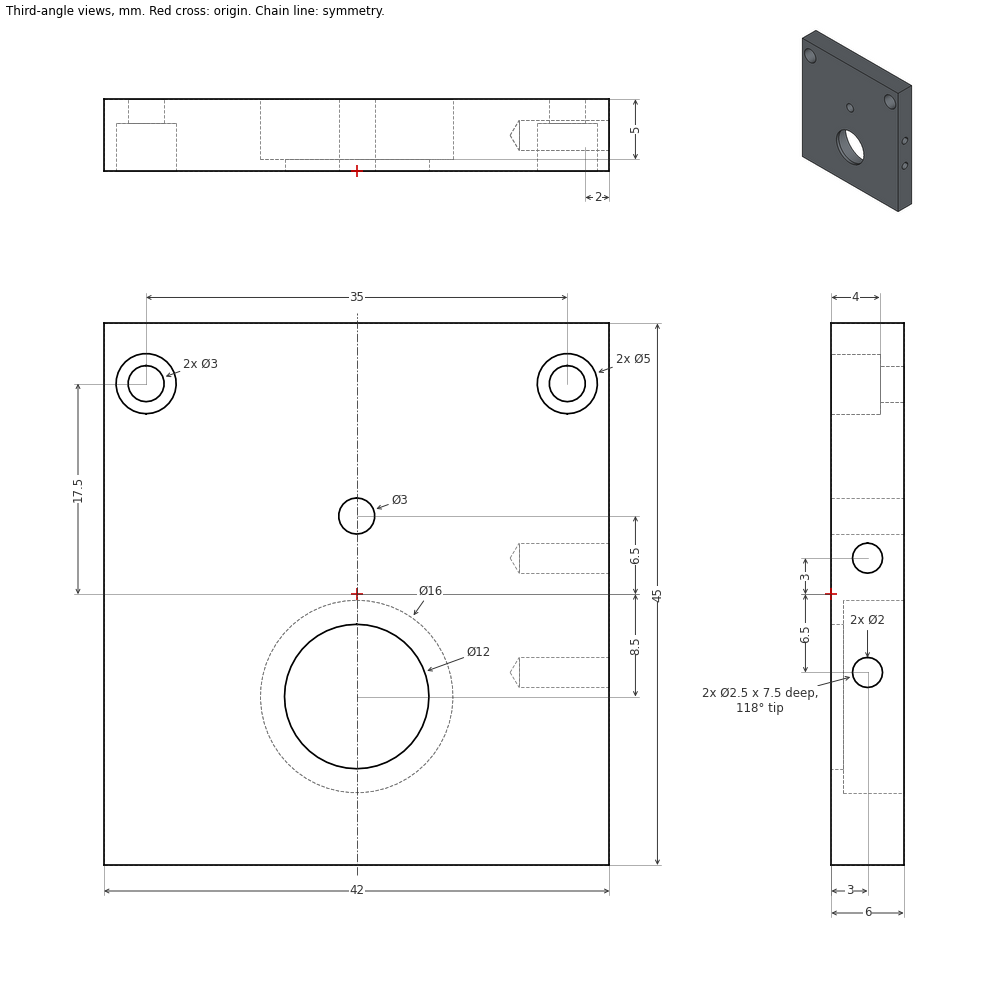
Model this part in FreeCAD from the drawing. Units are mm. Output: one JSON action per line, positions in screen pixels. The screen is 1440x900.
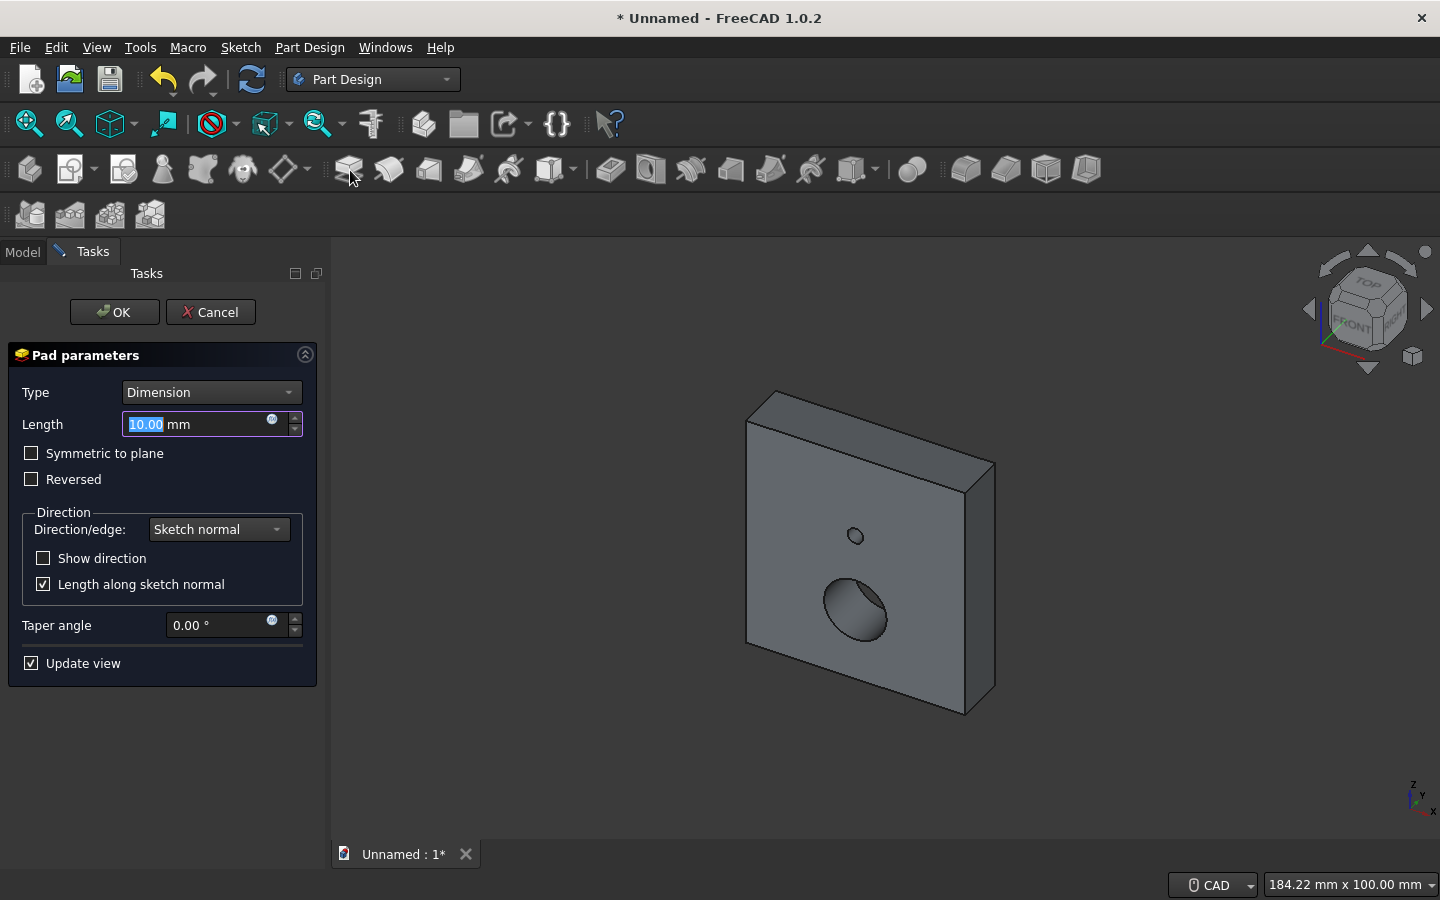
{"action": "type", "text": "6"}
{"action": "key", "text": "Tab"}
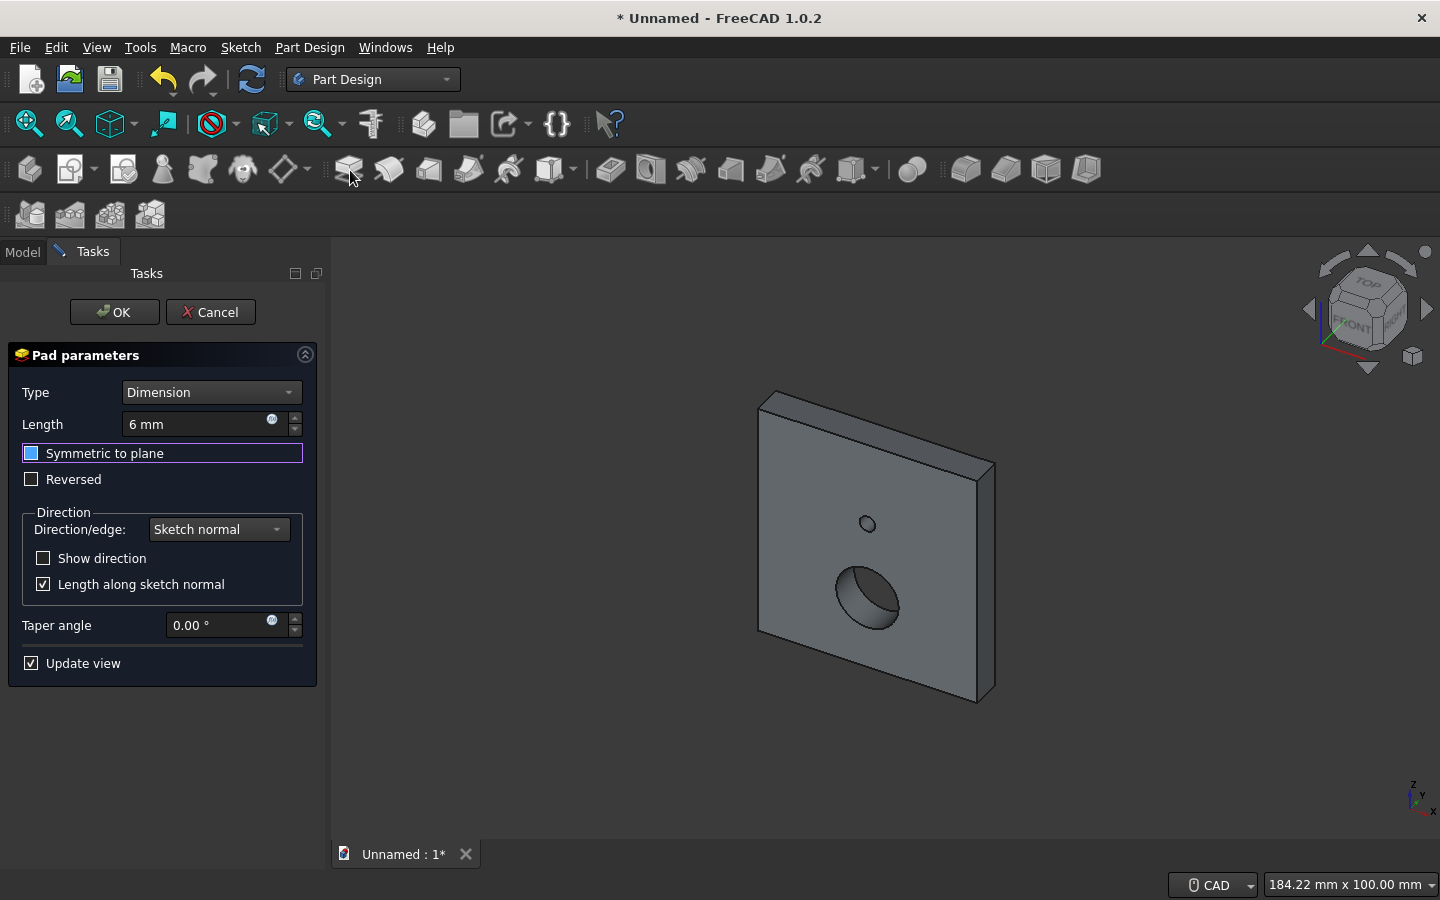
{"action": "left_click", "coordinate": [30, 479]}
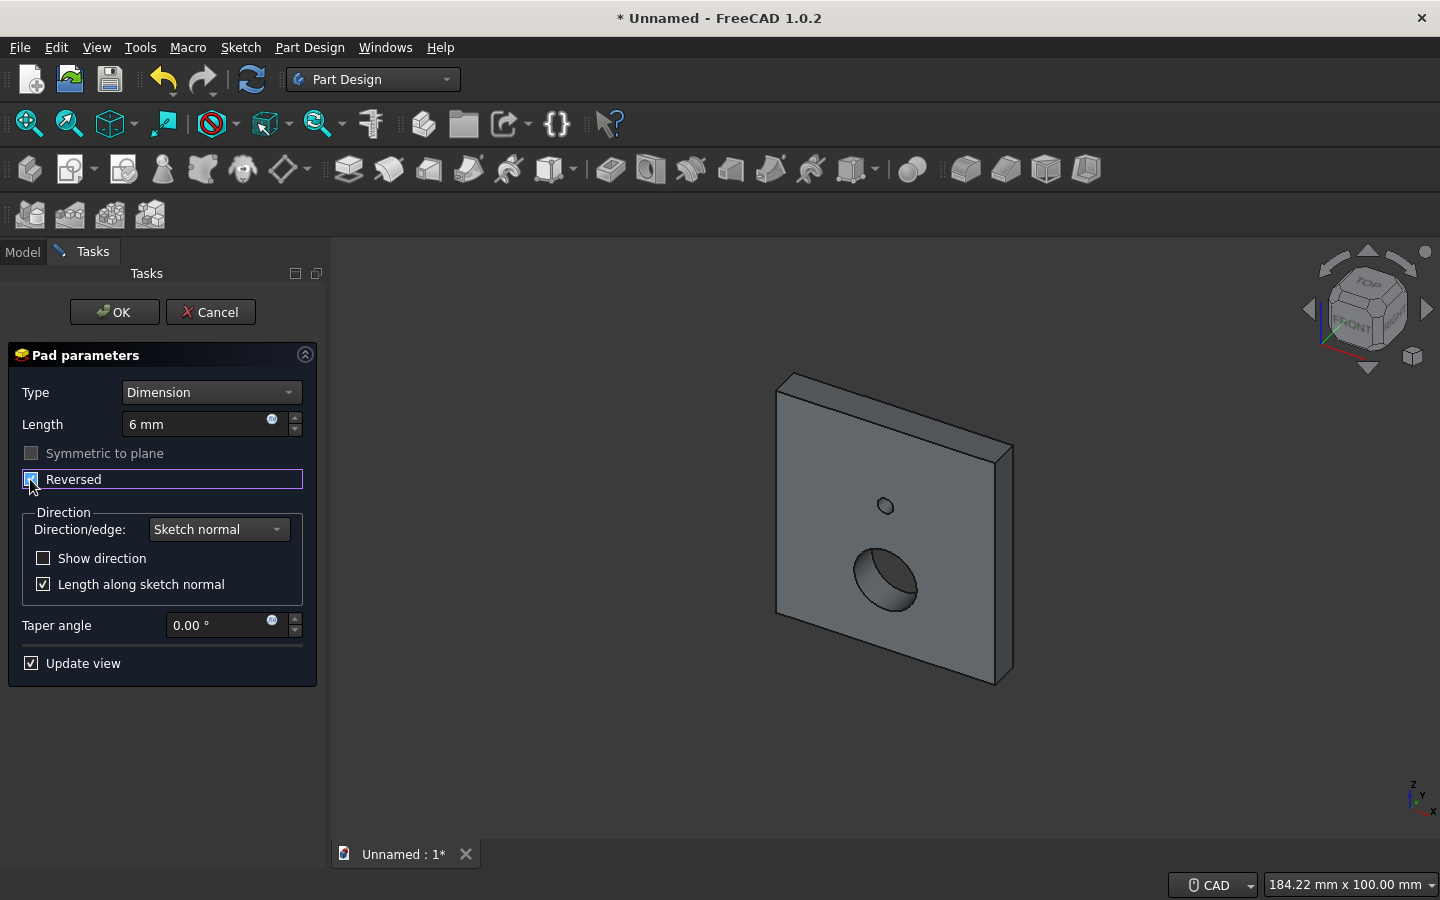
{"action": "left_click", "coordinate": [115, 312]}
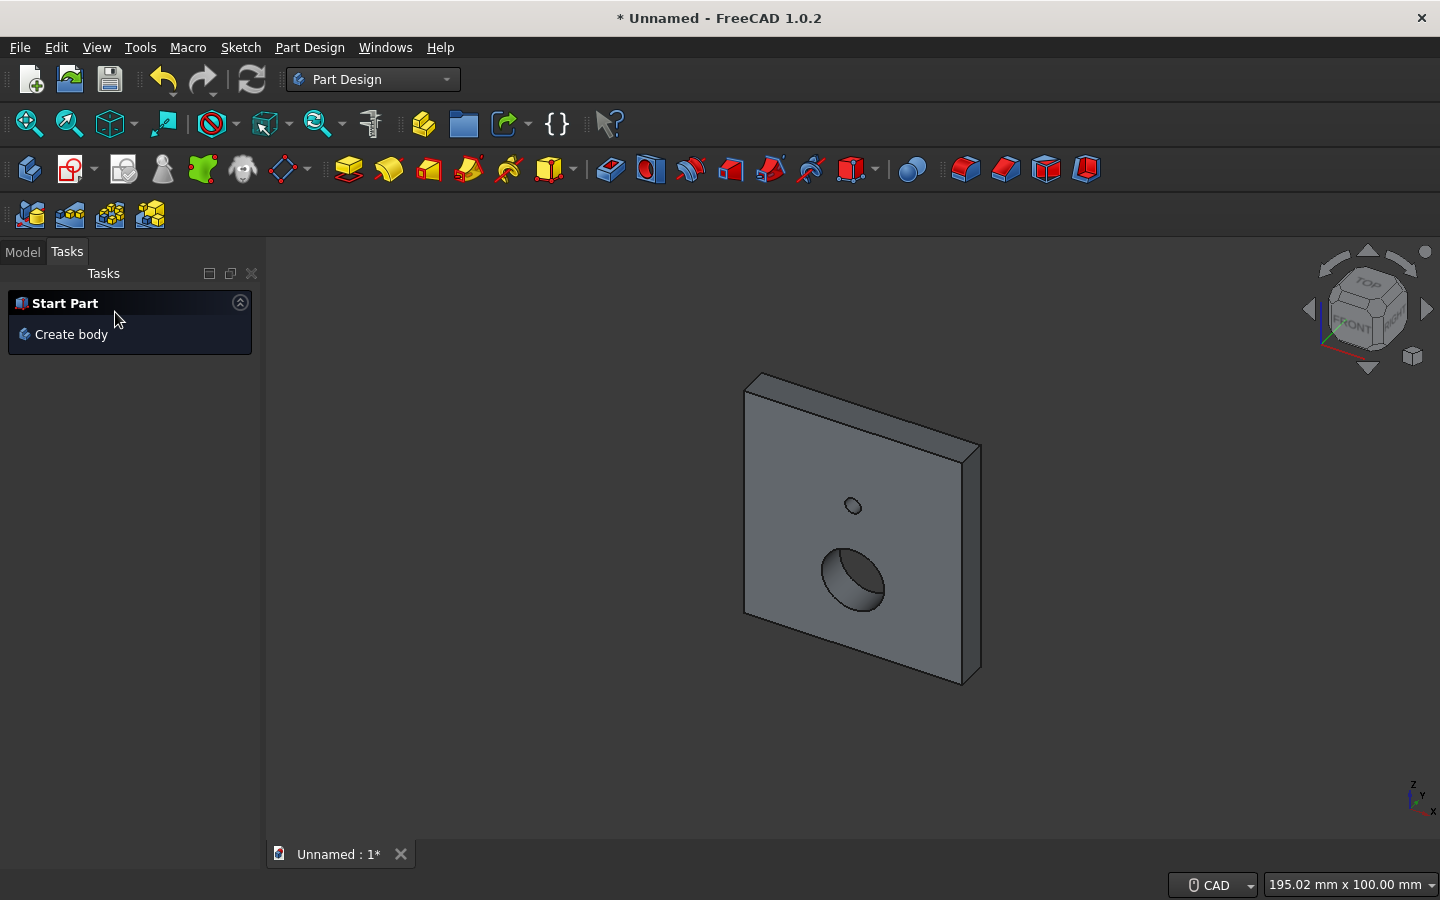
{"action": "key", "text": "4"}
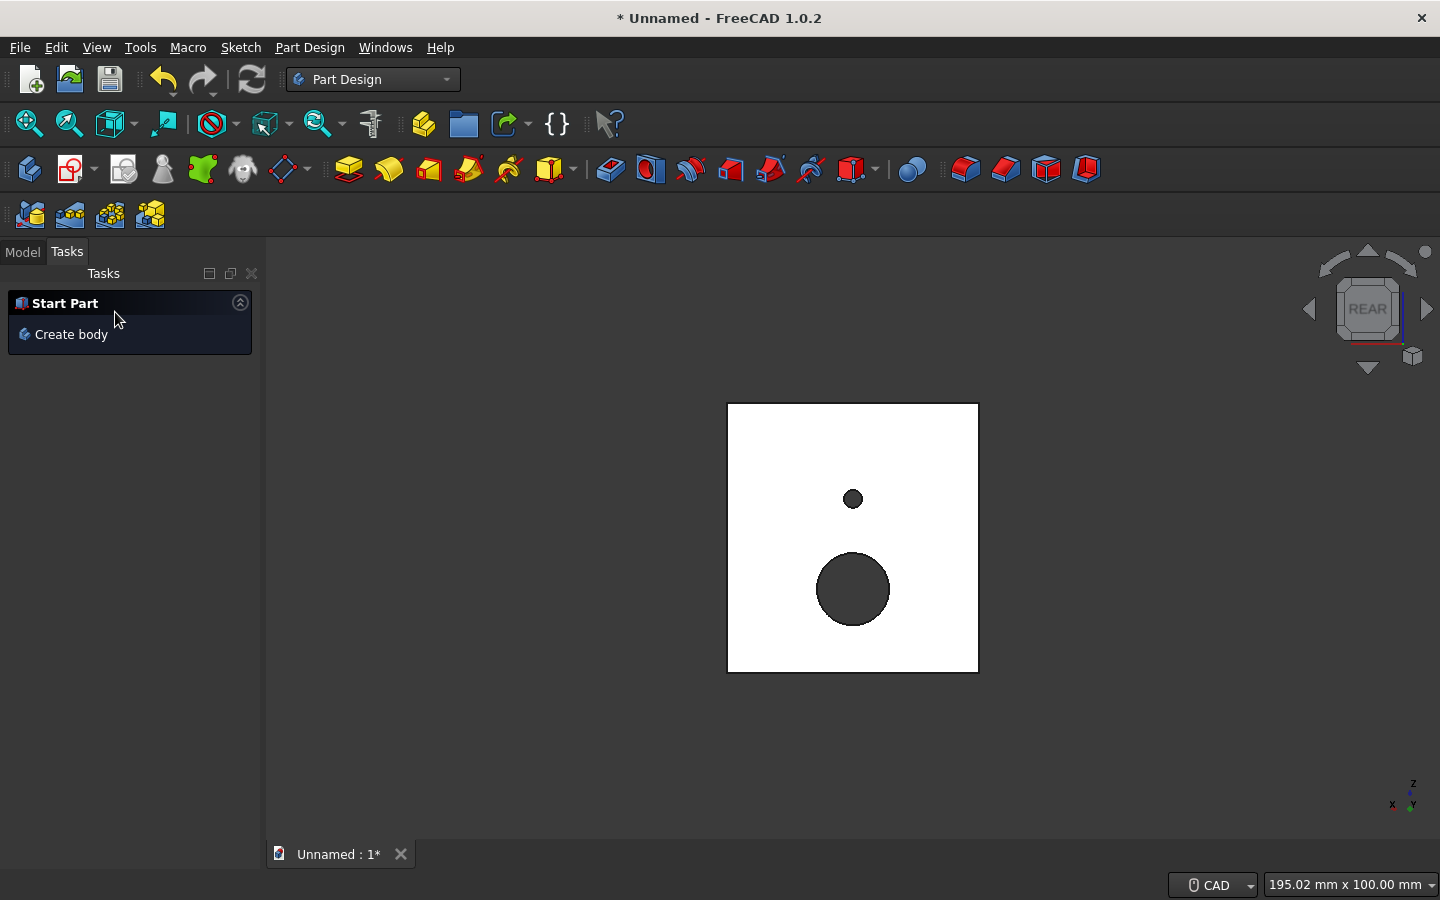
{"action": "key", "text": "v f"}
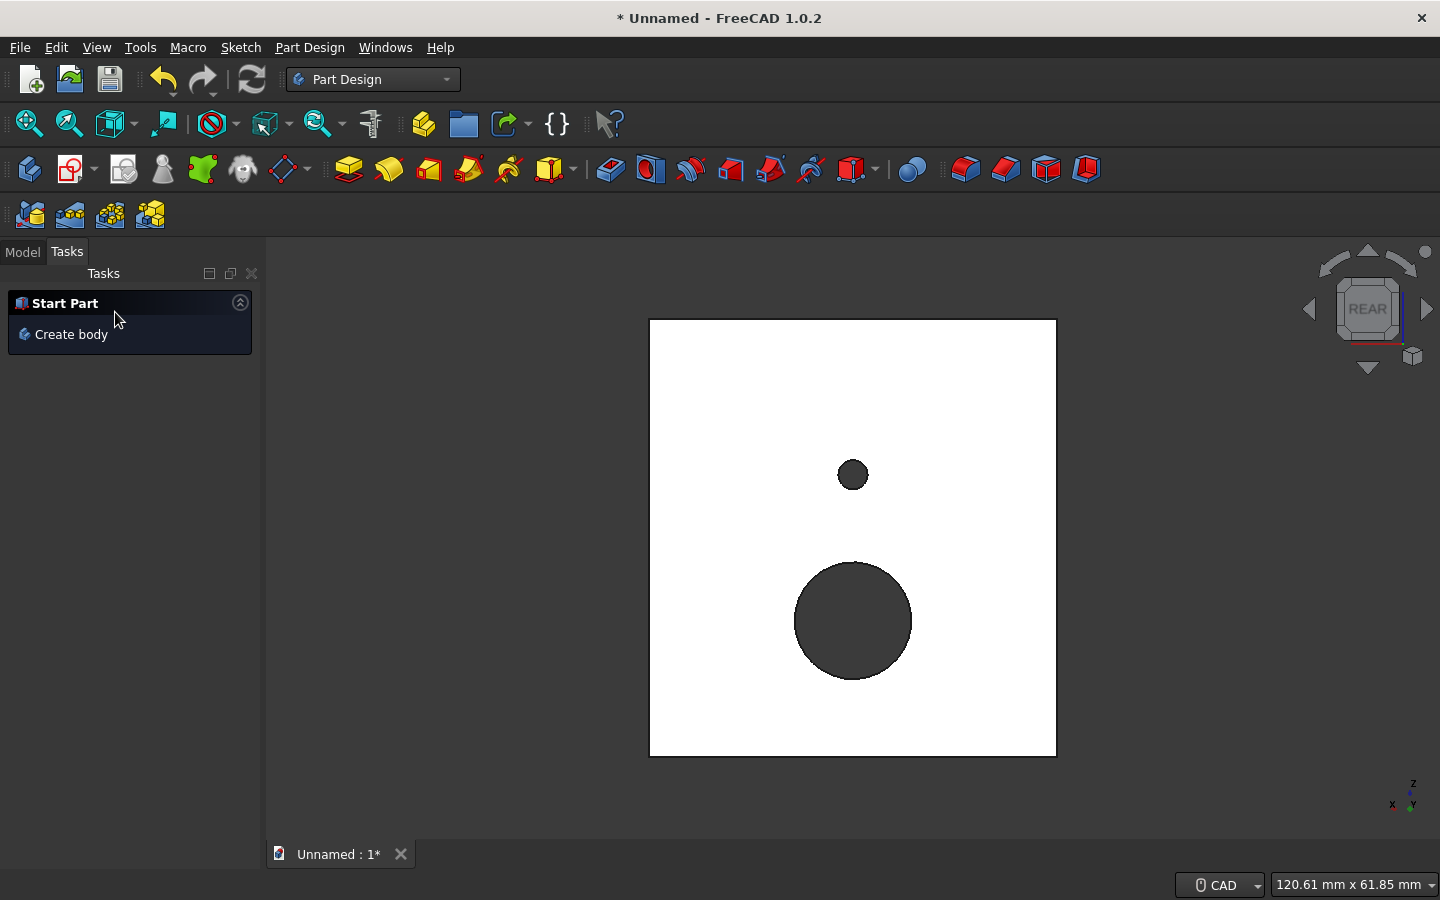
{"action": "left_click", "coordinate": [736, 412]}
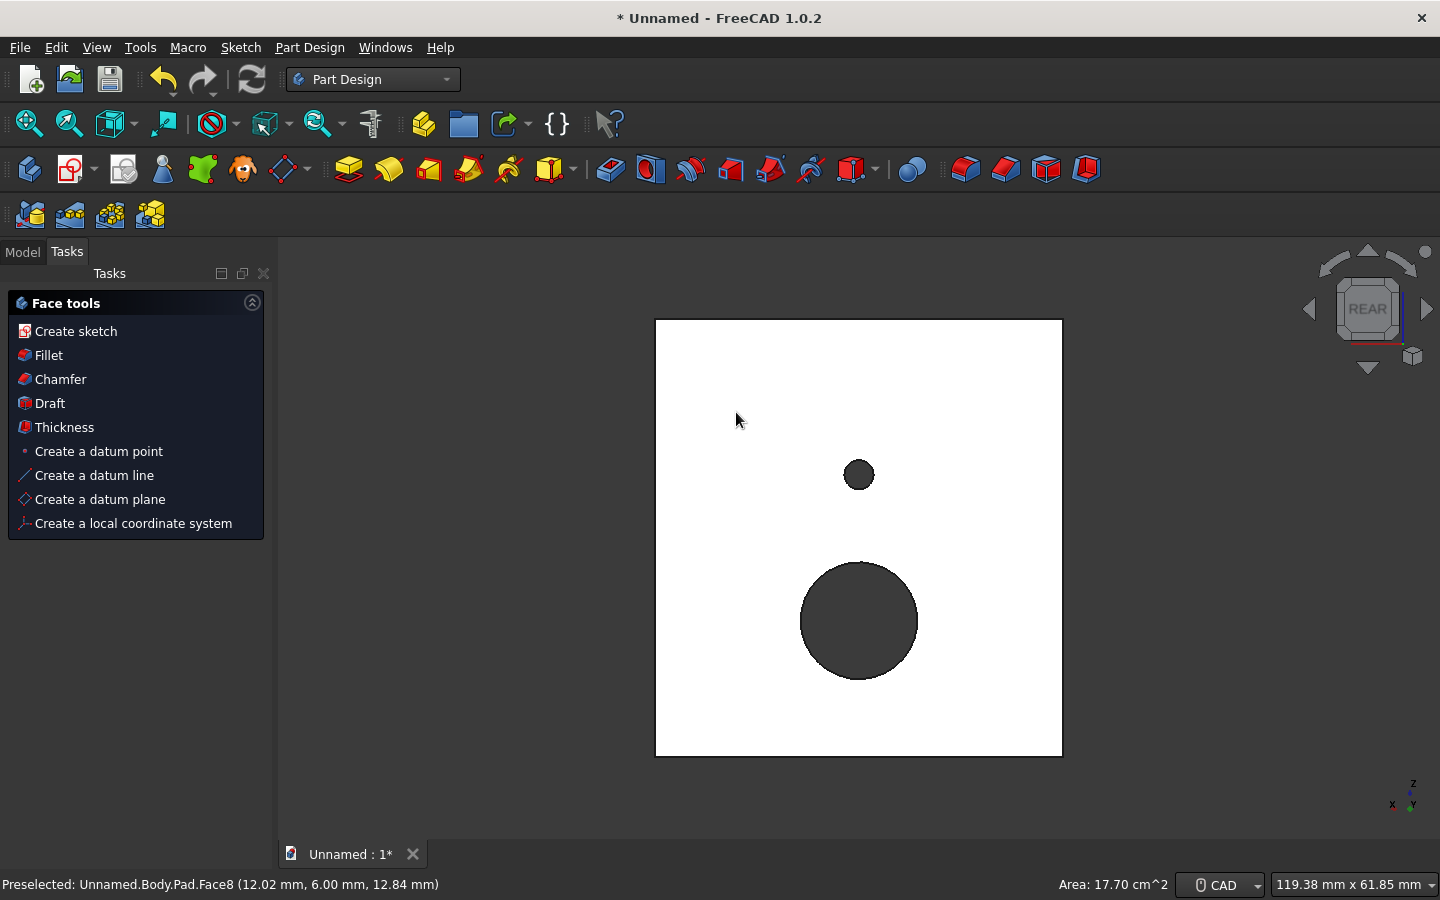
{"action": "left_click", "coordinate": [70, 170]}